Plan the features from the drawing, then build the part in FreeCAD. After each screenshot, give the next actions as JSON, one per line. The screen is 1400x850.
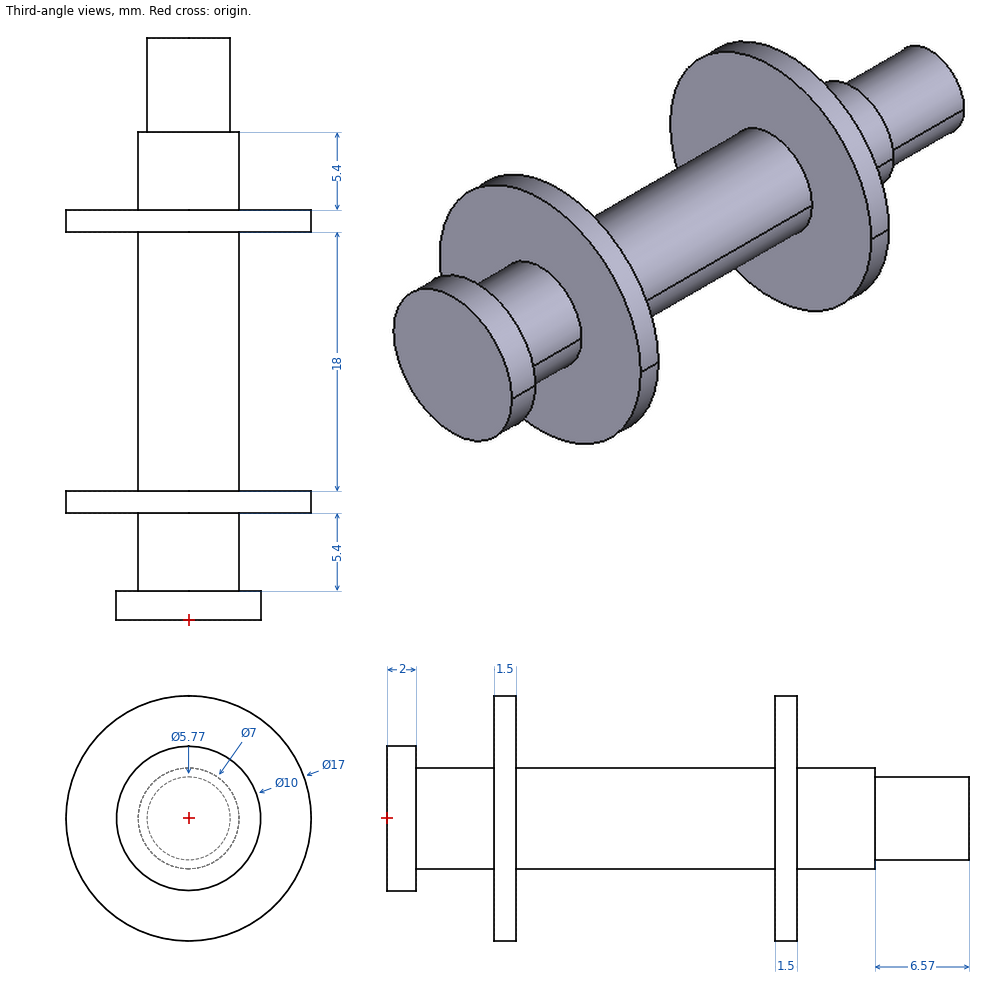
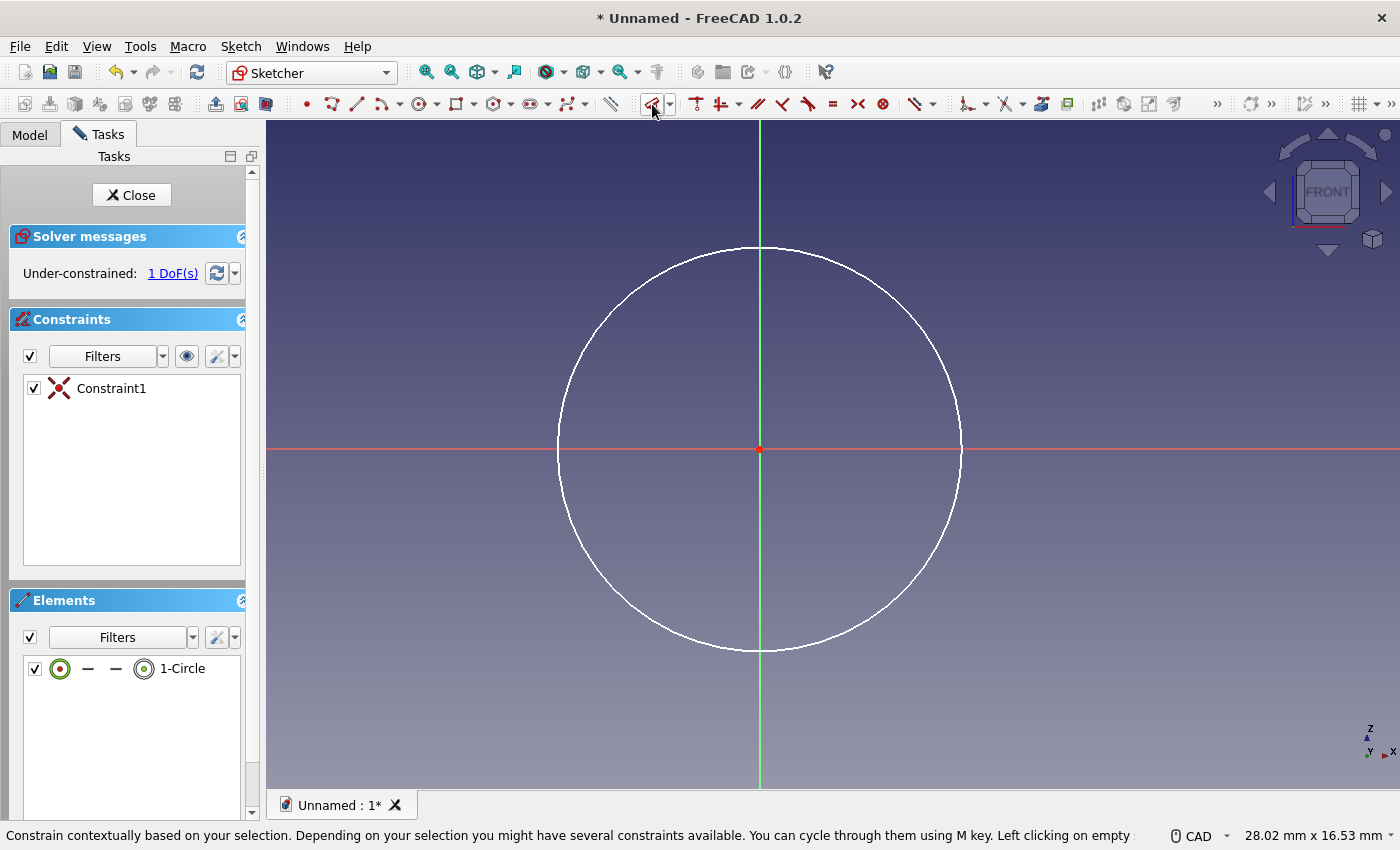
{"action": "left_click", "coordinate": [902, 306]}
{"action": "left_click", "coordinate": [925, 283]}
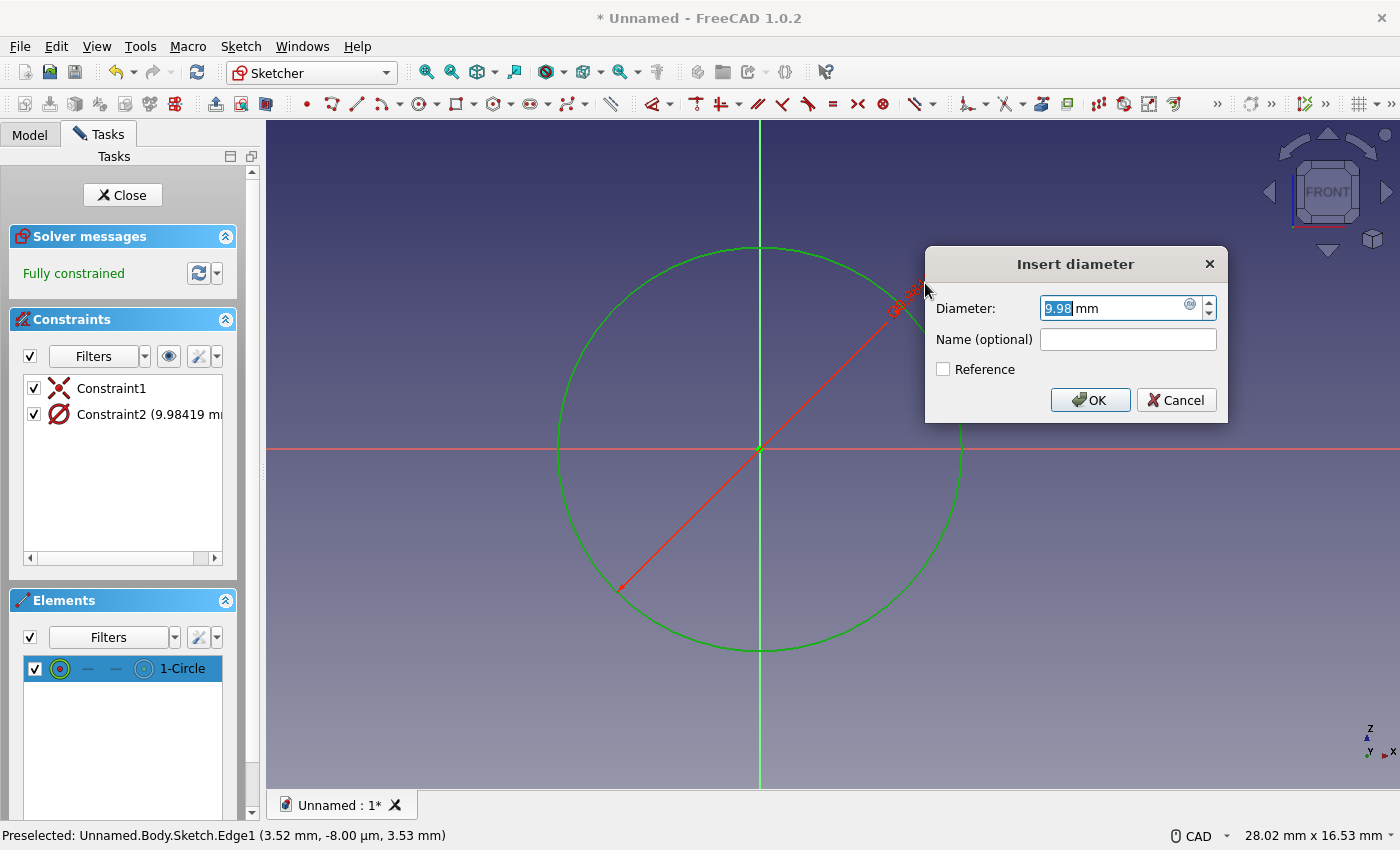
{"action": "type", "text": "10"}
{"action": "key", "text": "Return"}
{"action": "key", "text": "Escape"}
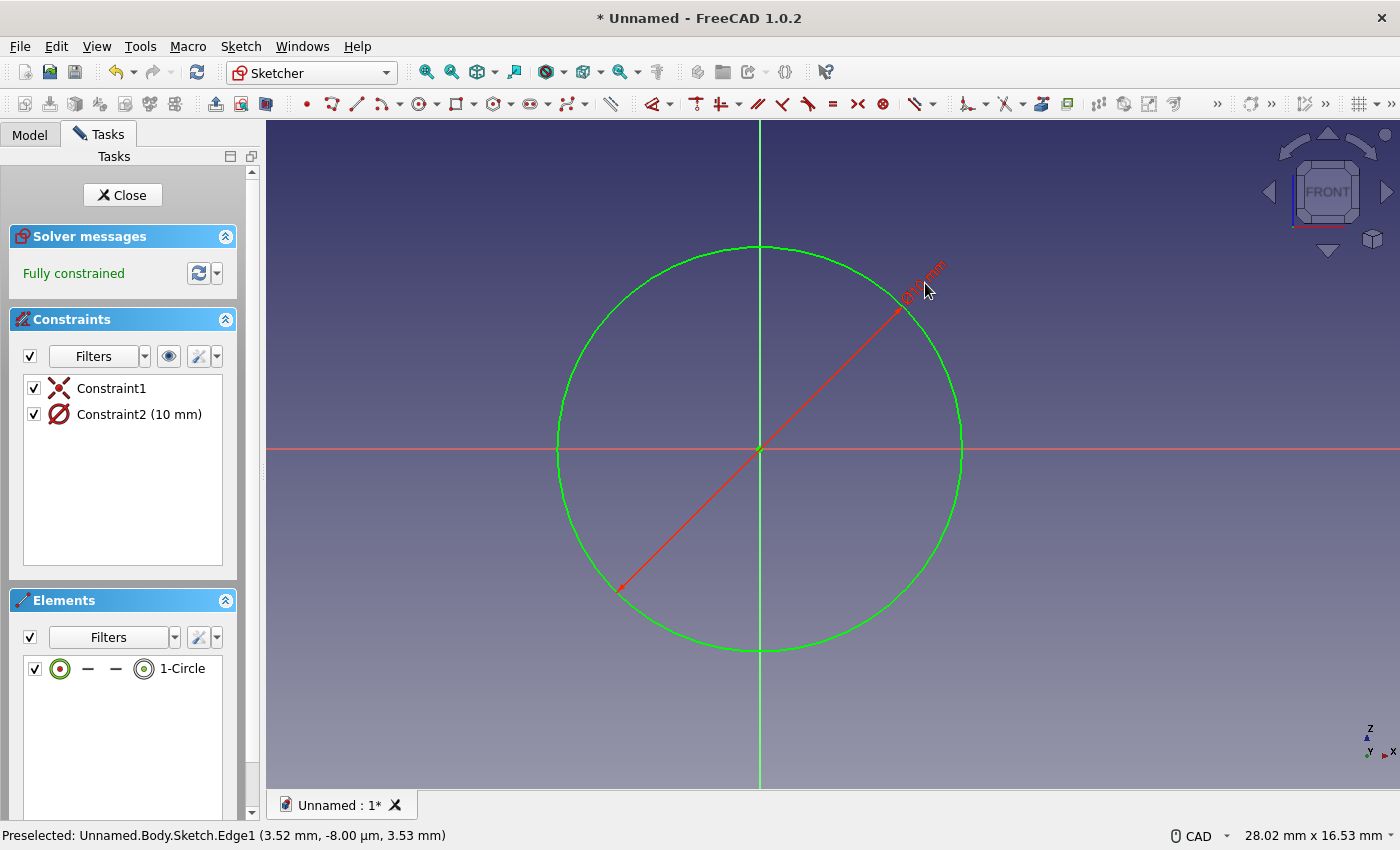
{"action": "left_click", "coordinate": [123, 195]}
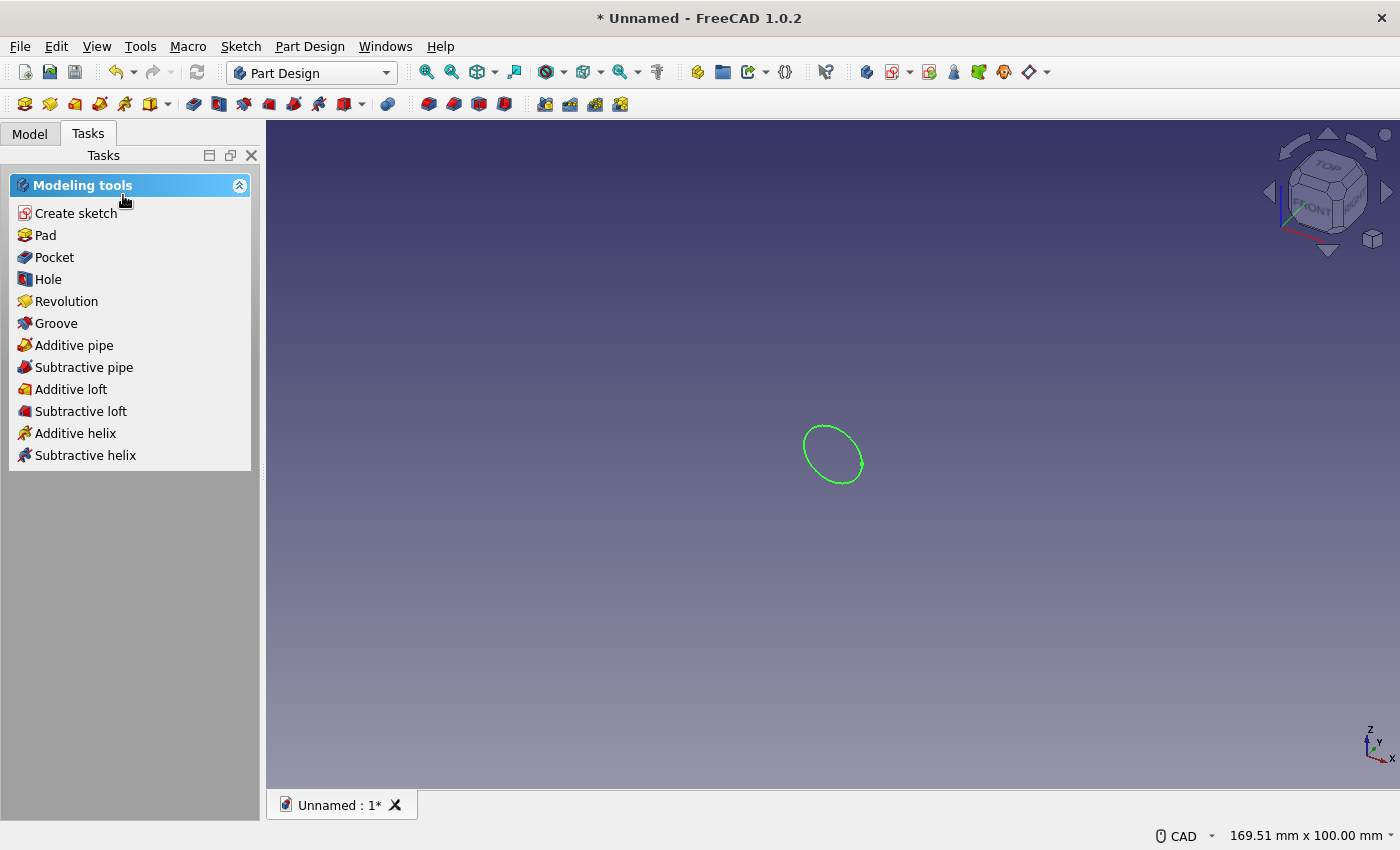
{"action": "left_click", "coordinate": [25, 104]}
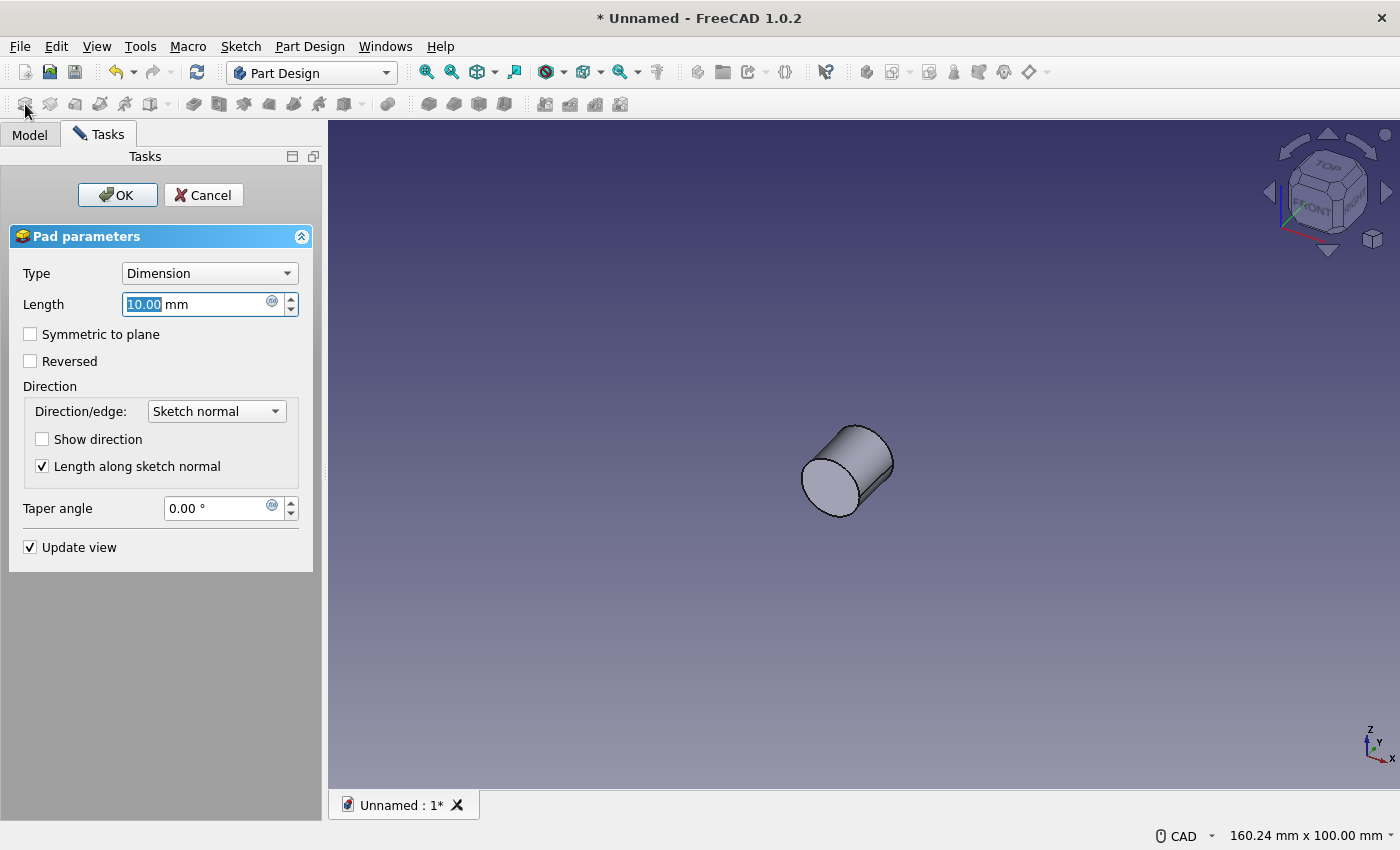
{"action": "type", "text": "2"}
{"action": "key", "text": "Tab"}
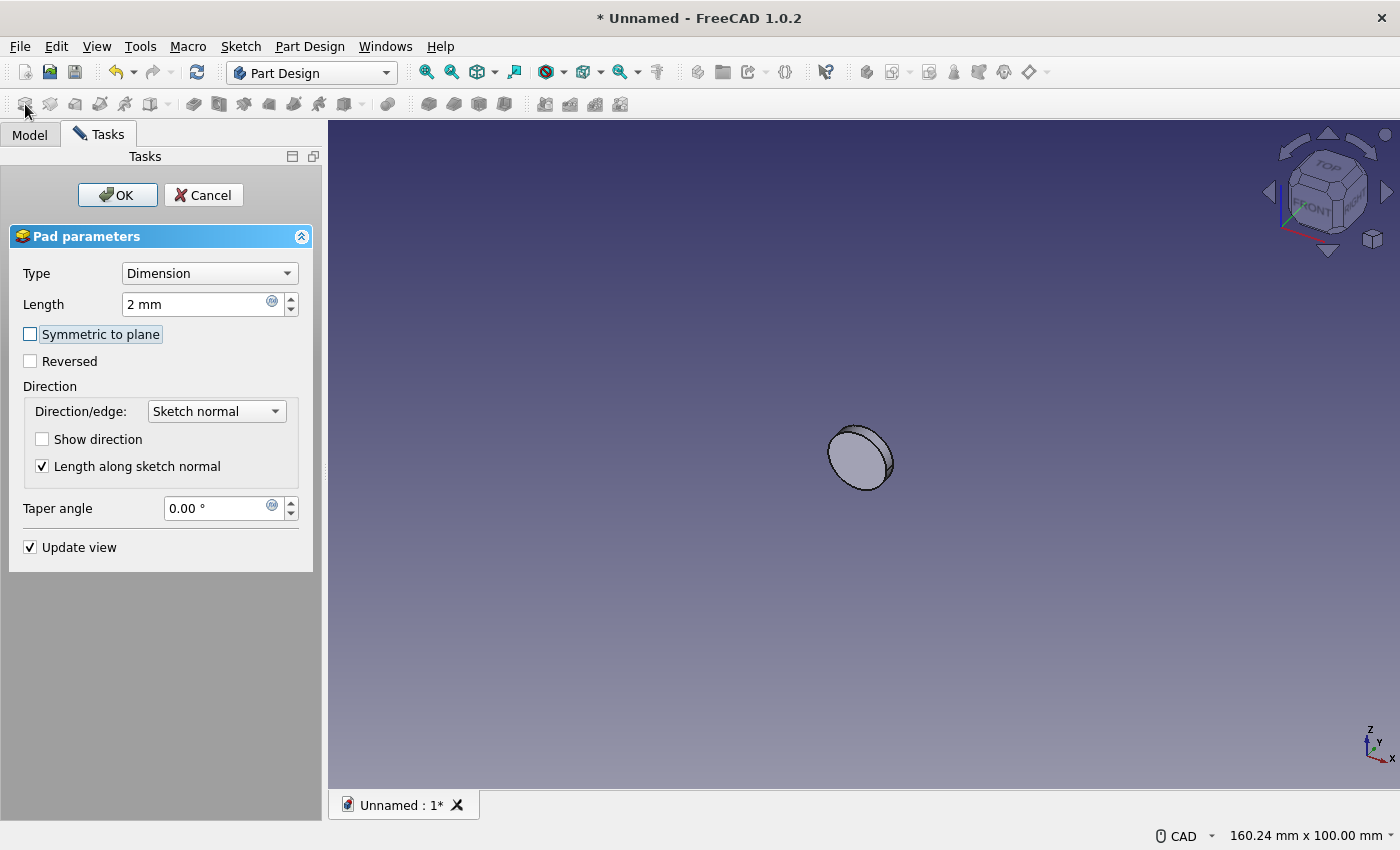
{"action": "left_click", "coordinate": [31, 361]}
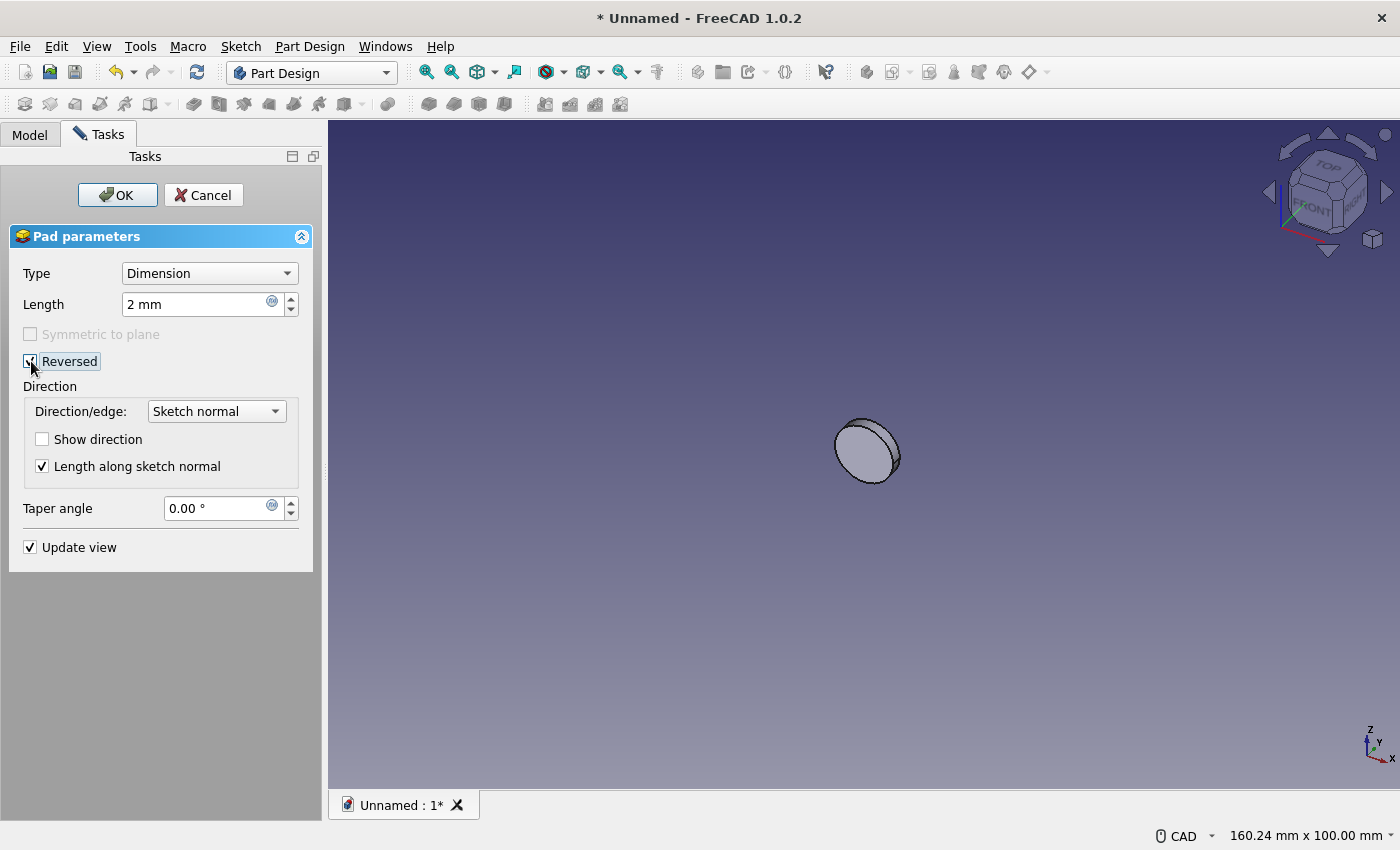
{"action": "left_click", "coordinate": [118, 195]}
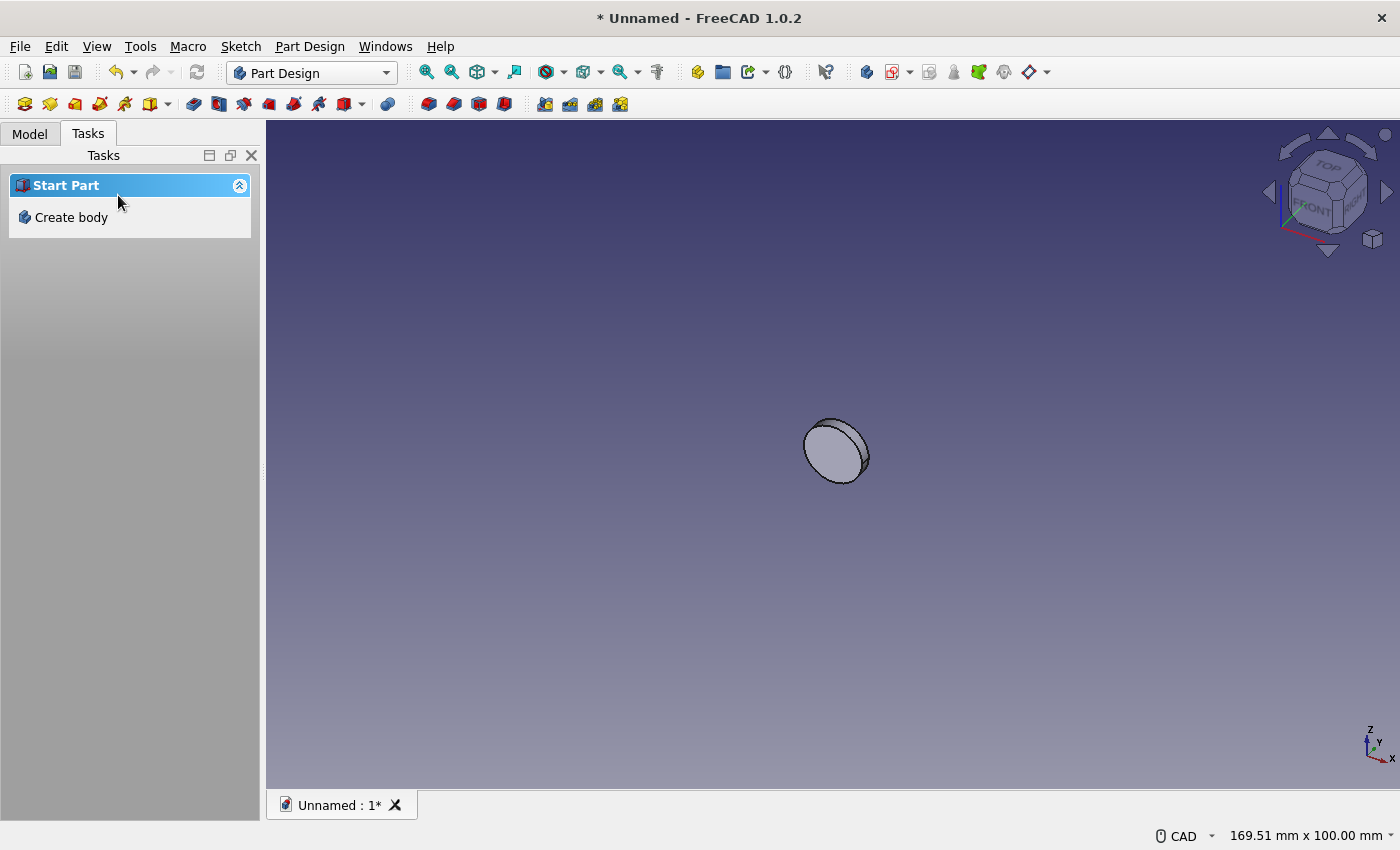
{"action": "left_click", "coordinate": [427, 72]}